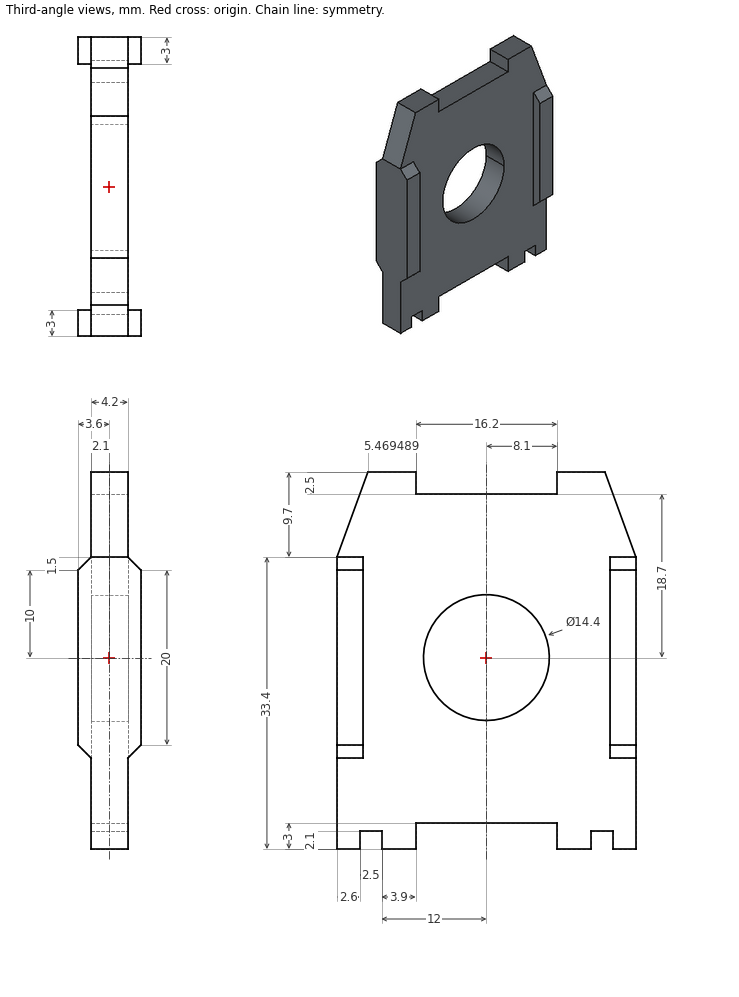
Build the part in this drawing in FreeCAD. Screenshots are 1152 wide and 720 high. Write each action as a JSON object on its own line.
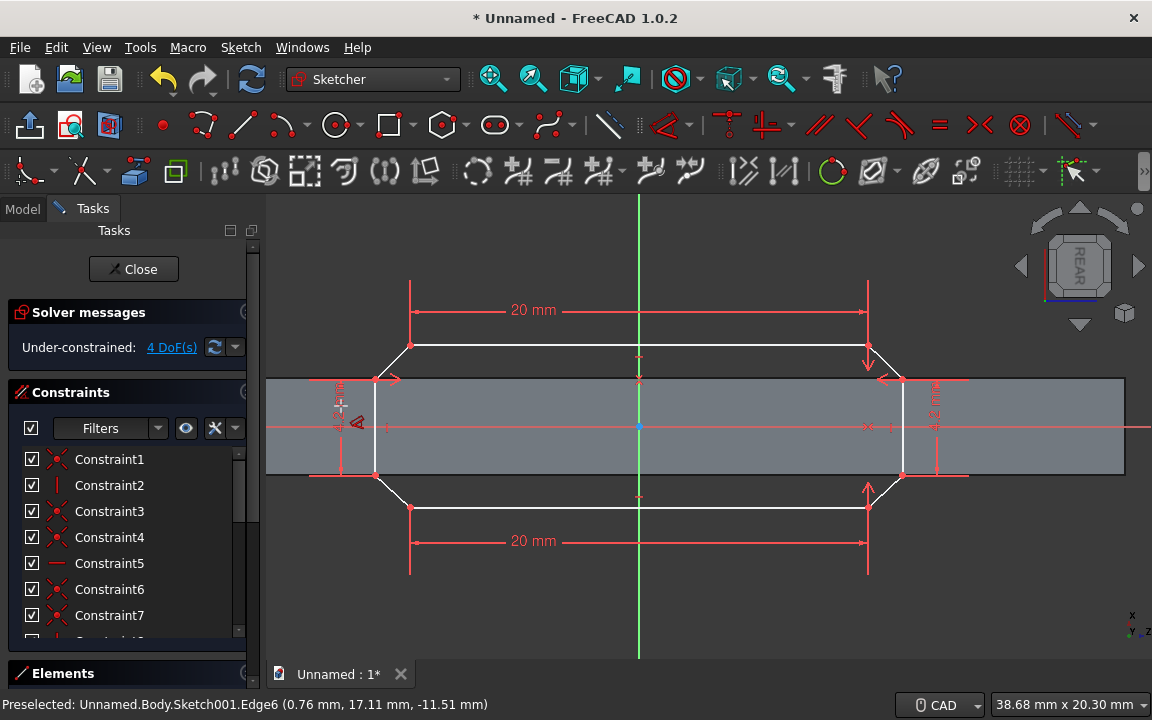
{"action": "left_click", "coordinate": [868, 508]}
{"action": "left_click", "coordinate": [754, 542]}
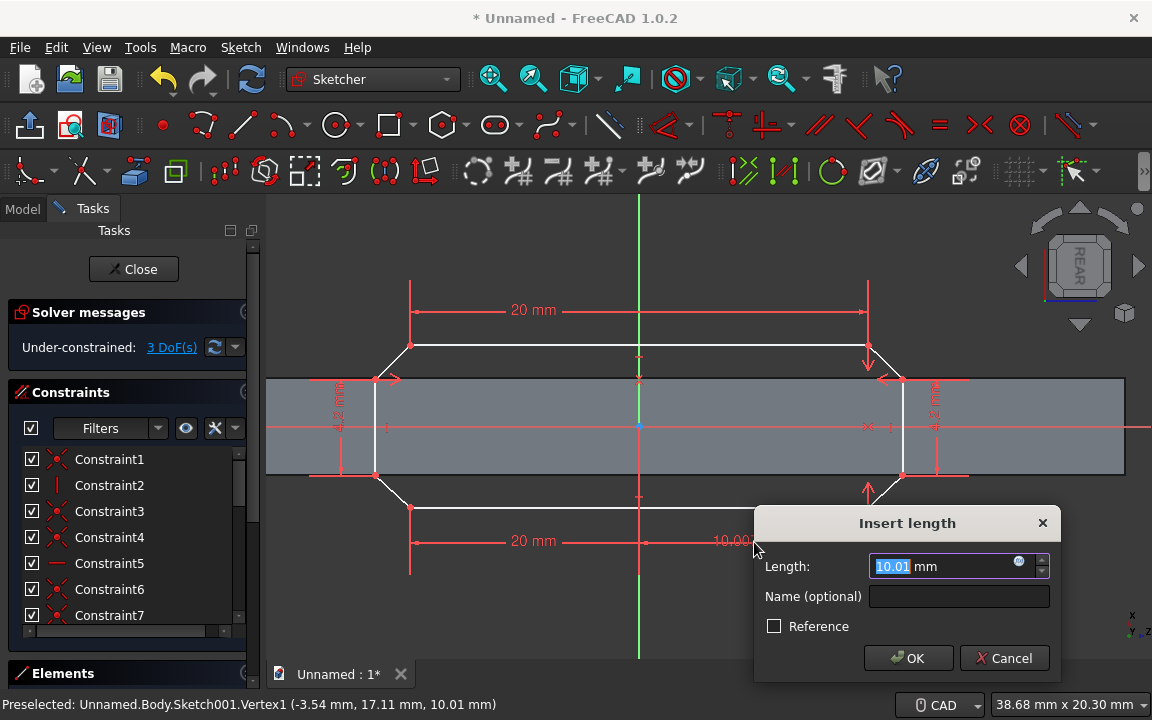
{"action": "type", "text": "10"}
{"action": "key", "text": "Return"}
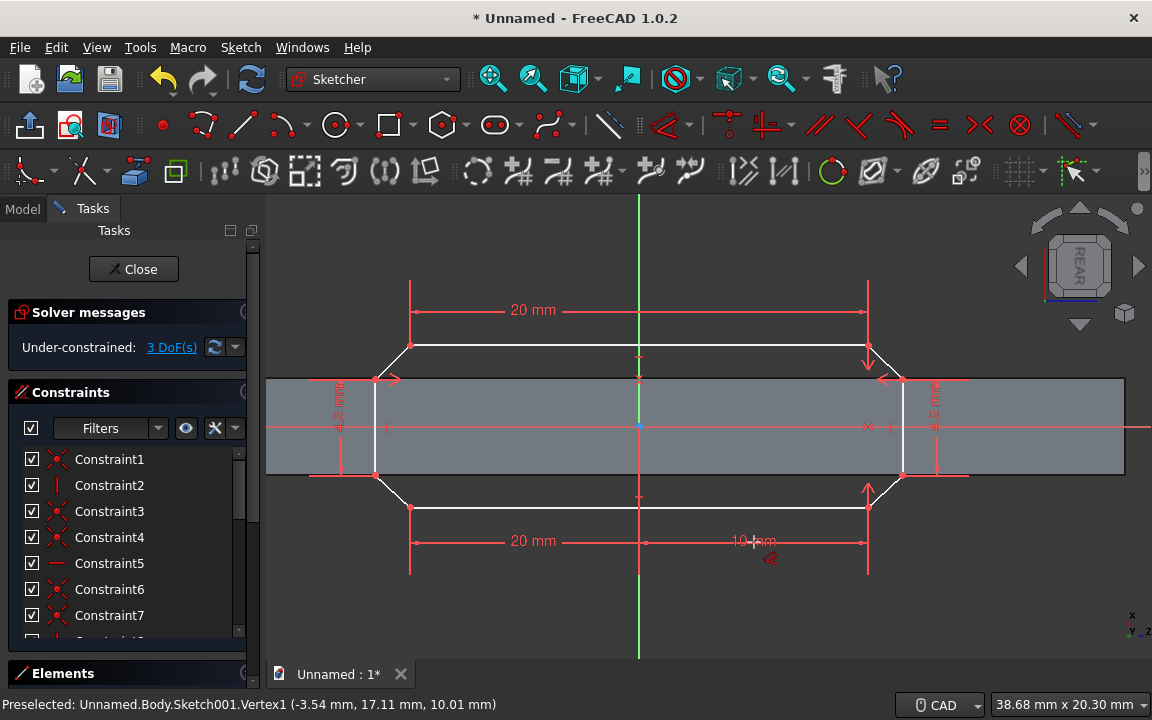
{"action": "left_click", "coordinate": [868, 508]}
{"action": "left_click", "coordinate": [902, 495]}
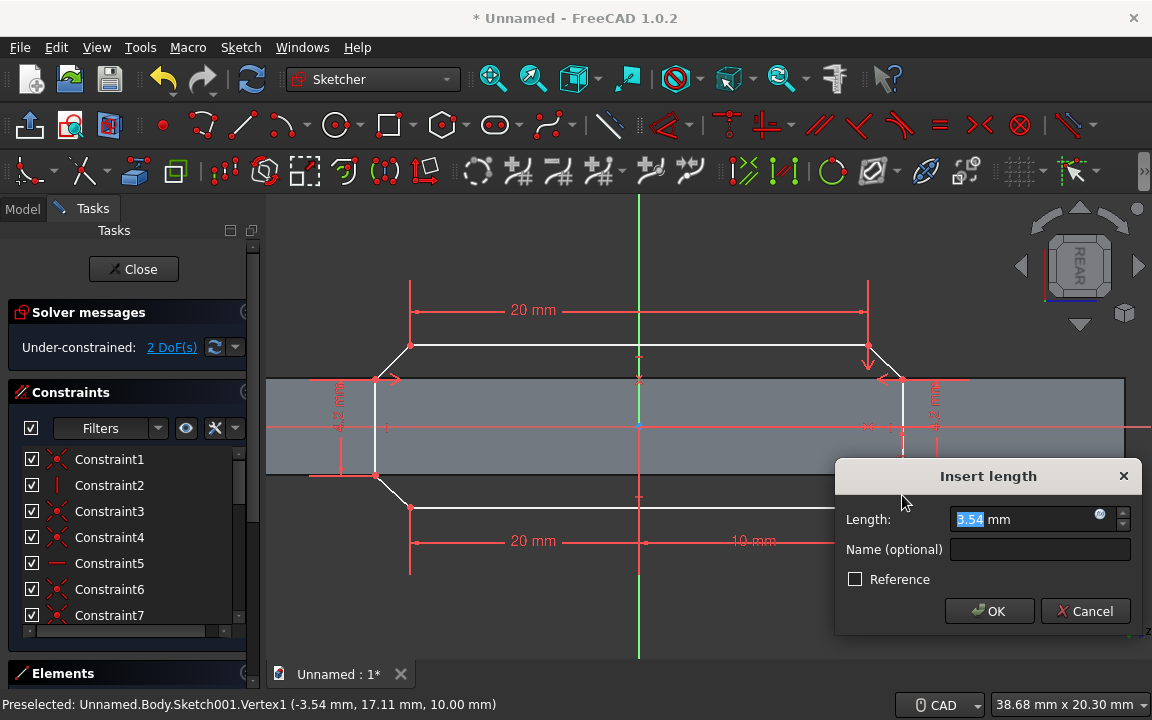
{"action": "type", "text": "3.6"}
{"action": "key", "text": "Return"}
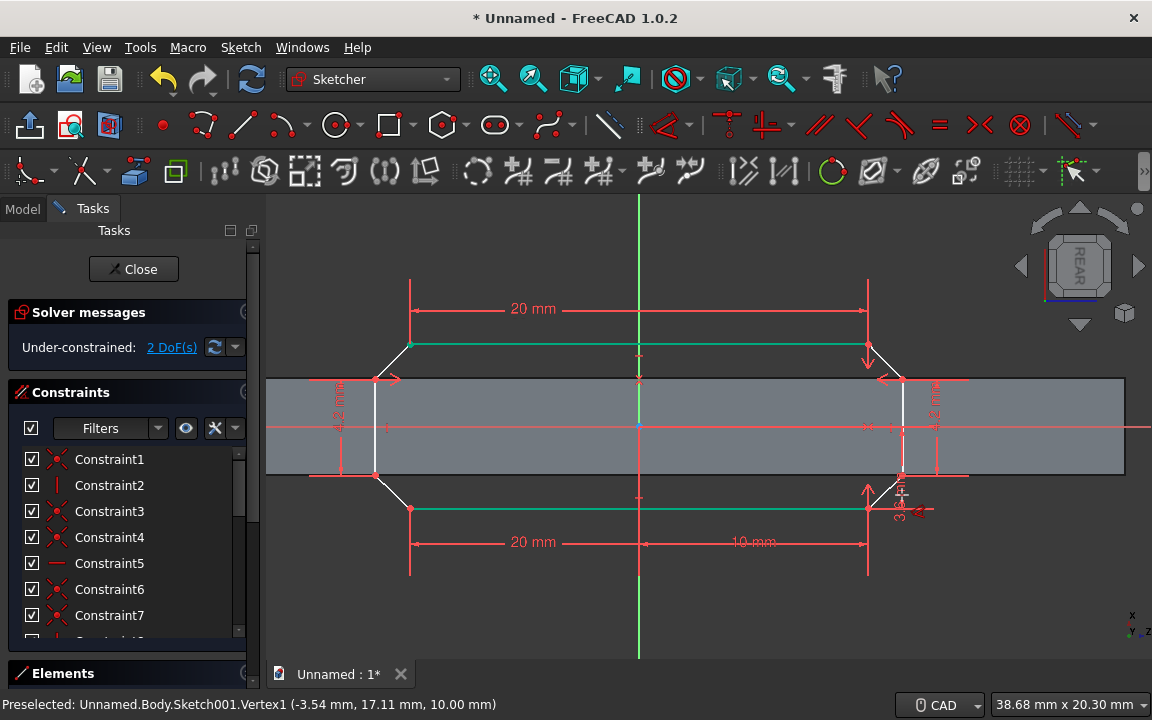
{"action": "left_click", "coordinate": [903, 476]}
{"action": "left_click", "coordinate": [937, 451]}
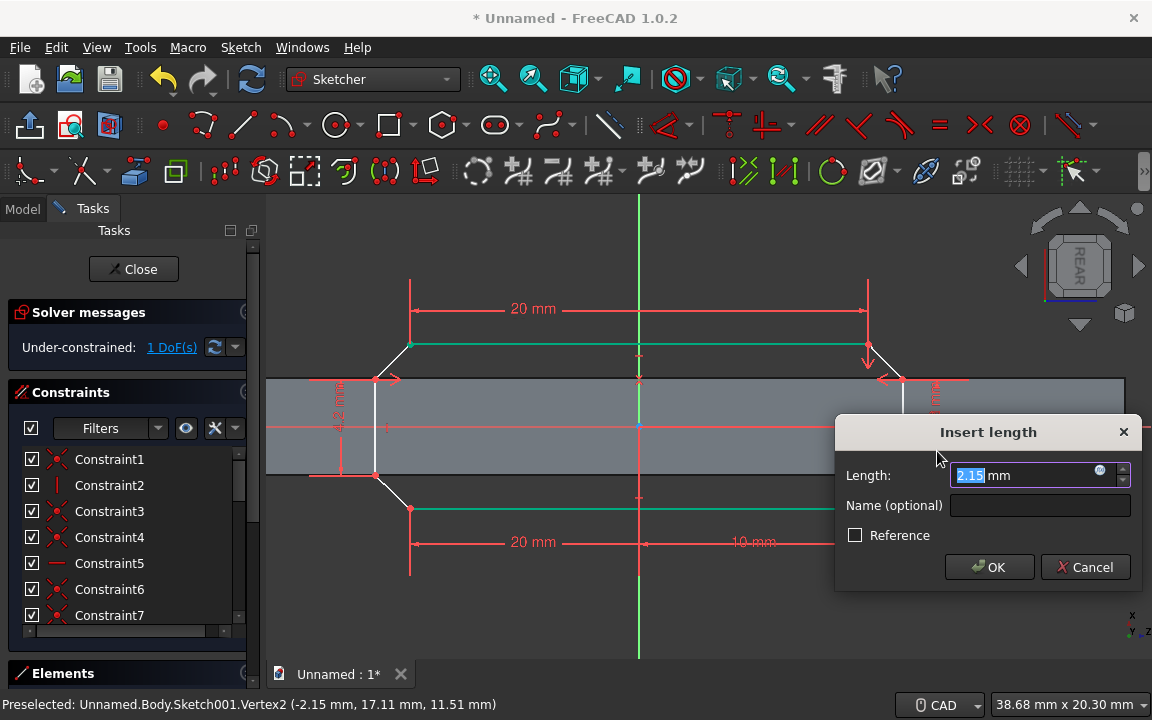
{"action": "type", "text": "2.1"}
{"action": "key", "text": "Return"}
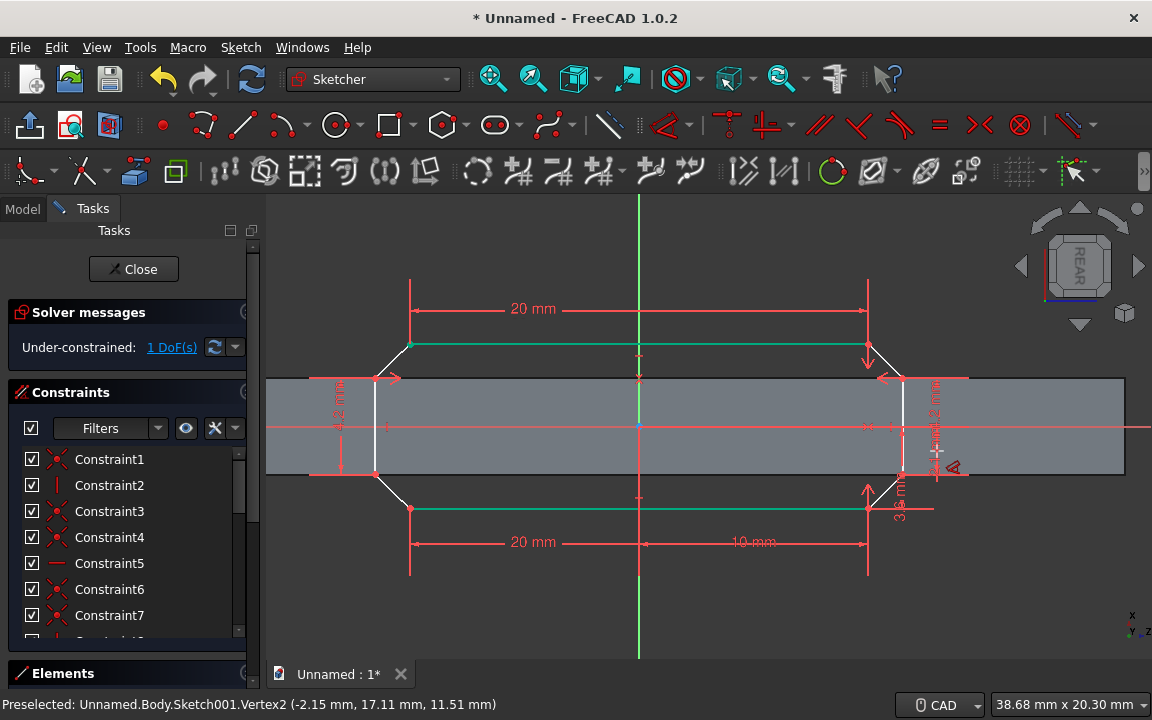
{"action": "left_click", "coordinate": [879, 499]}
{"action": "left_click", "coordinate": [885, 543]}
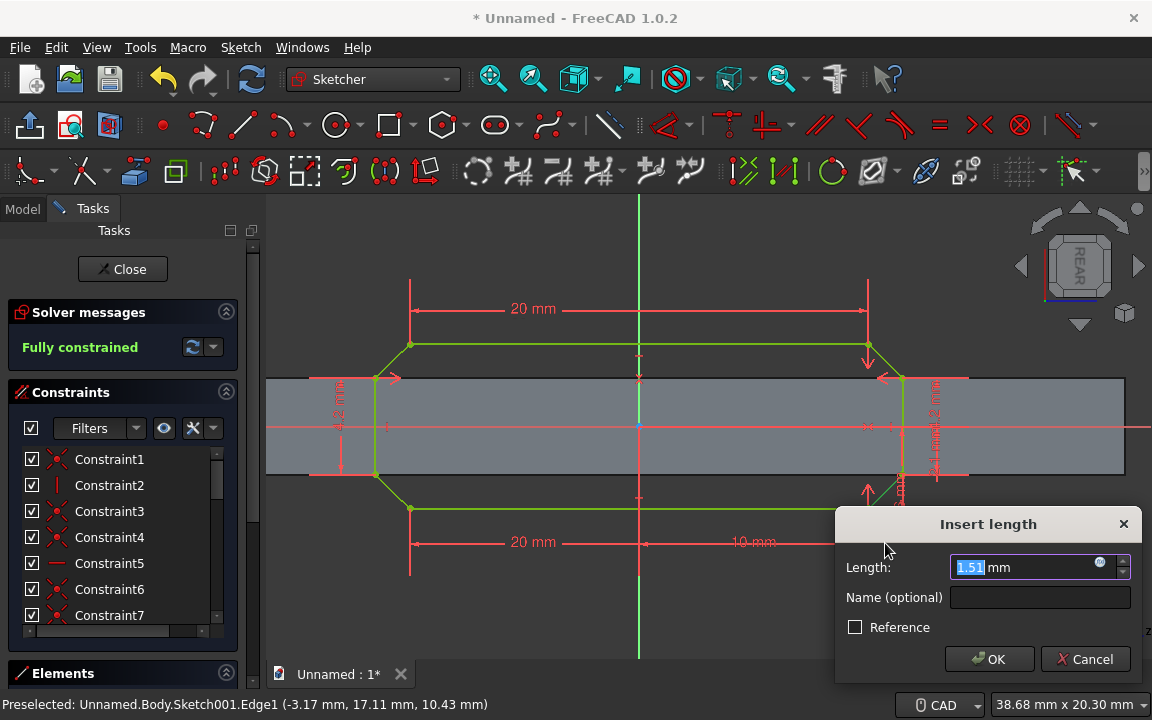
{"action": "type", "text": "1.5"}
{"action": "key", "text": "Return"}
{"action": "key", "text": "Escape"}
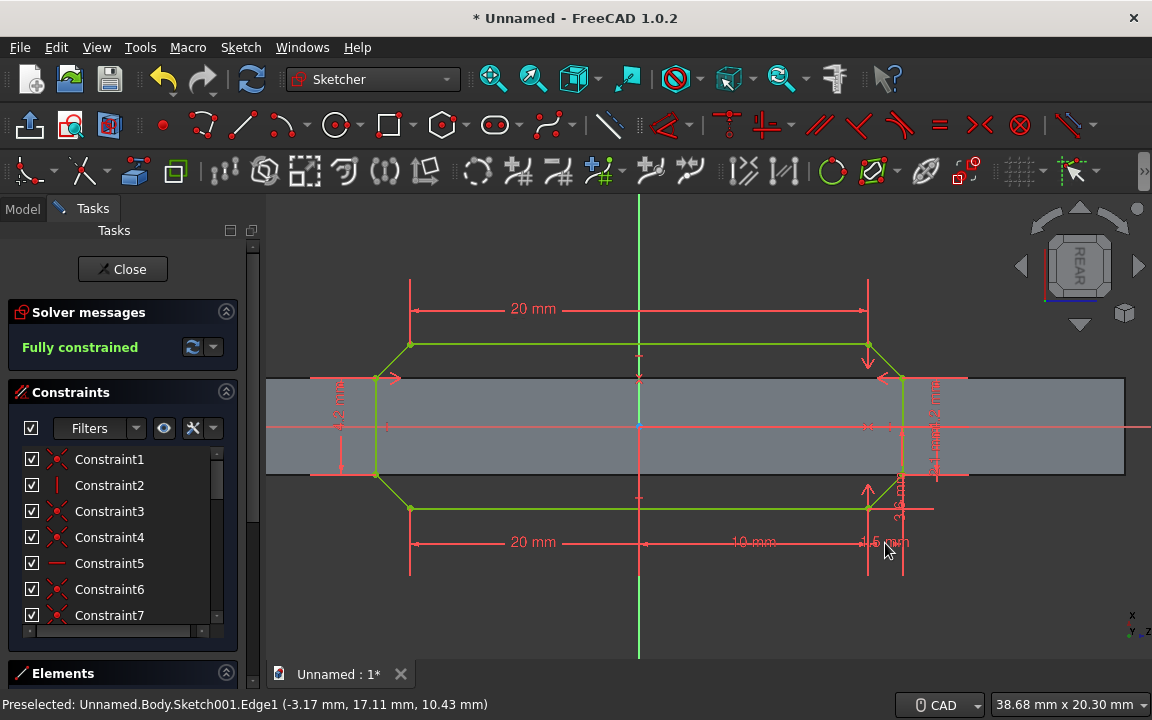
{"action": "left_click", "coordinate": [123, 269]}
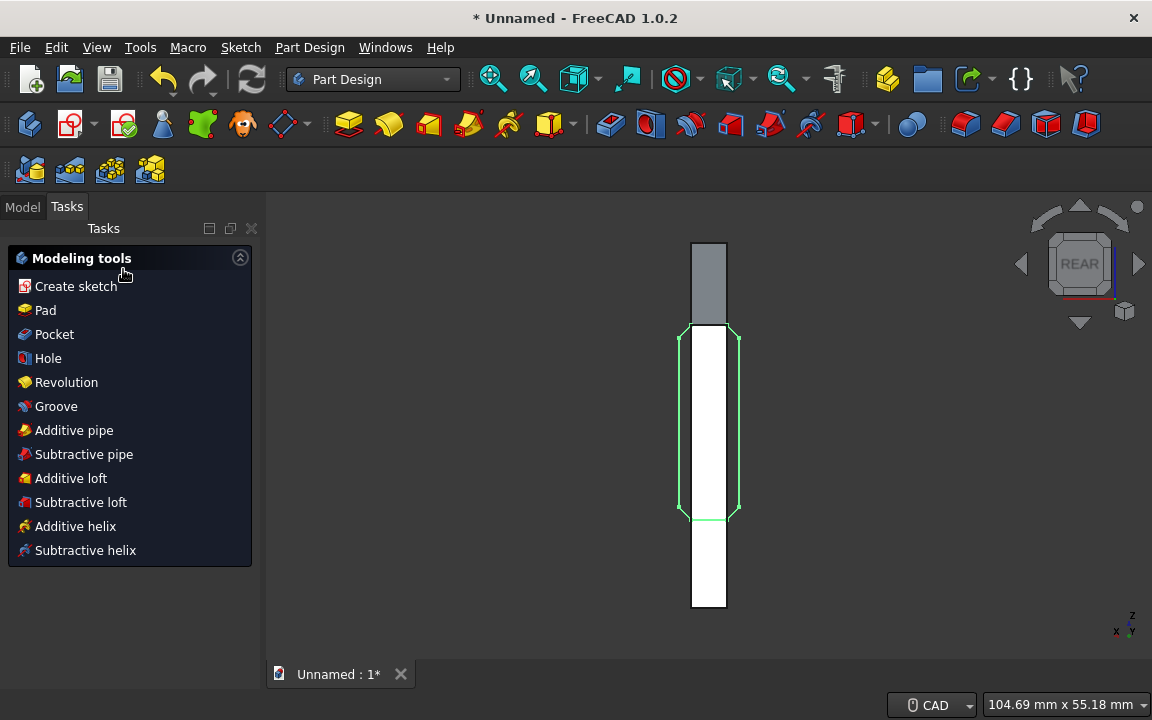
{"action": "left_click", "coordinate": [350, 124]}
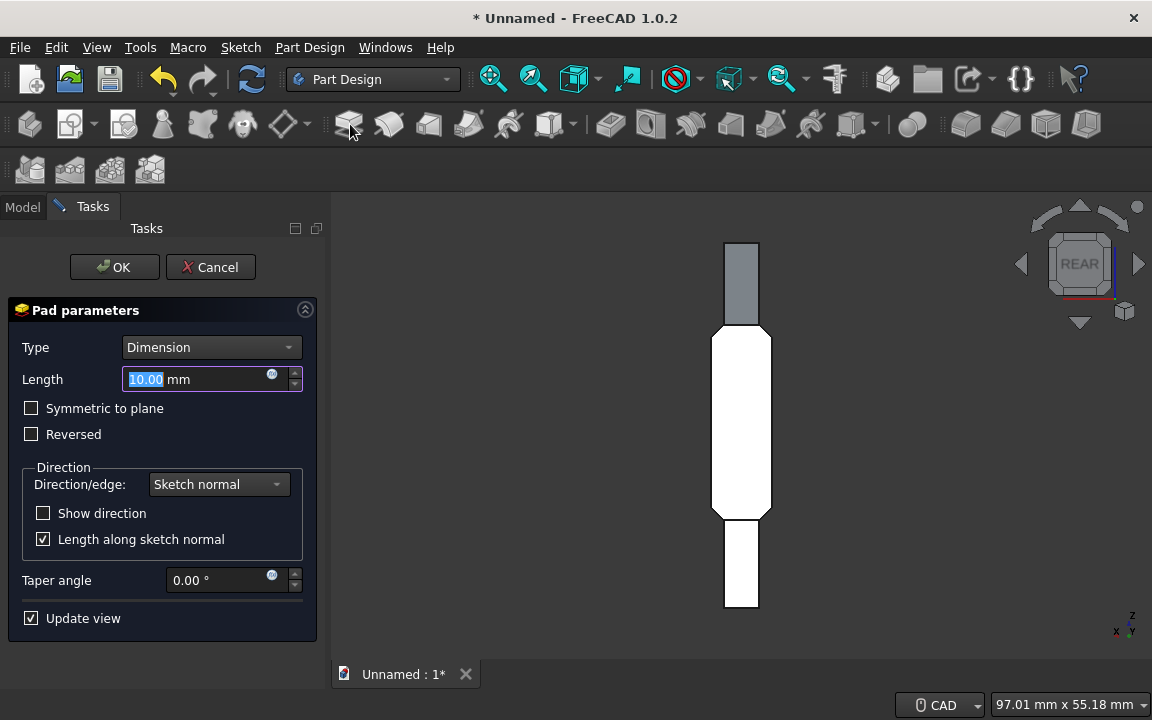
{"action": "type", "text": "3"}
{"action": "key", "text": "Tab"}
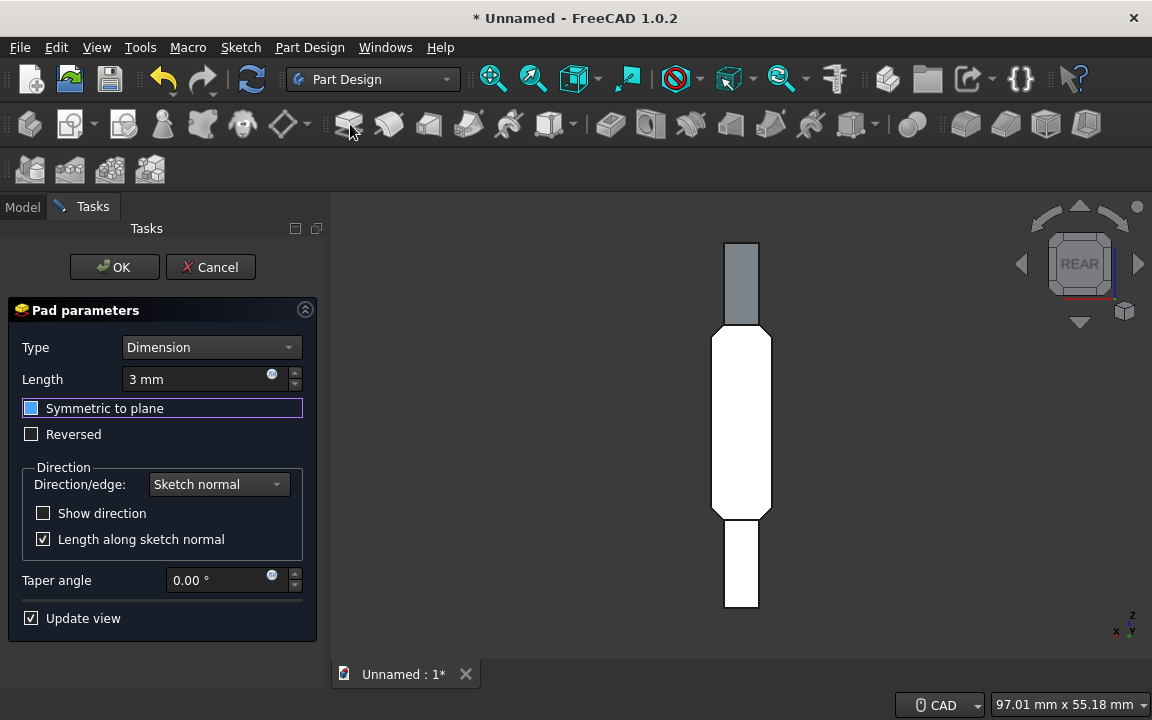
{"action": "left_click", "coordinate": [30, 434]}